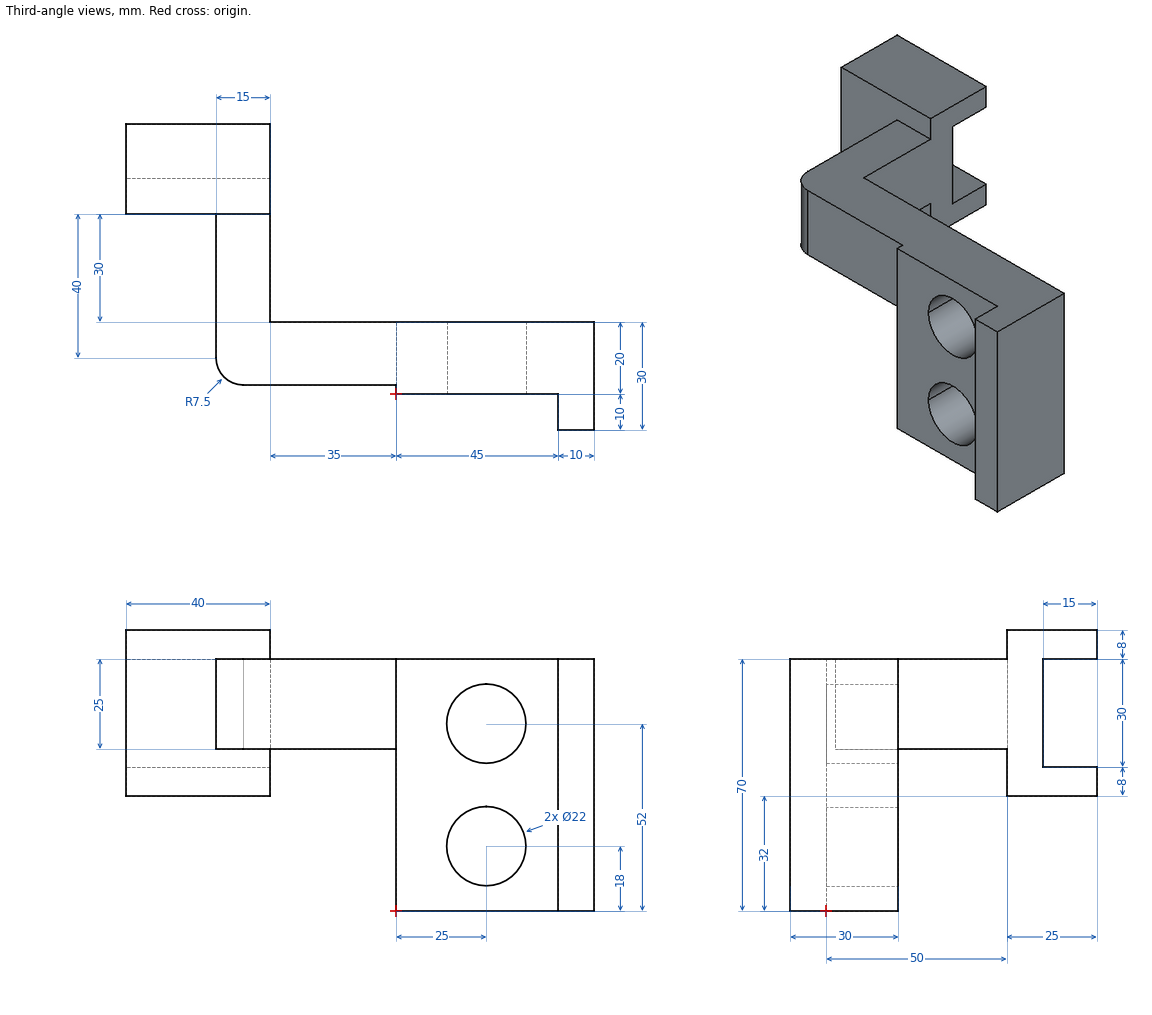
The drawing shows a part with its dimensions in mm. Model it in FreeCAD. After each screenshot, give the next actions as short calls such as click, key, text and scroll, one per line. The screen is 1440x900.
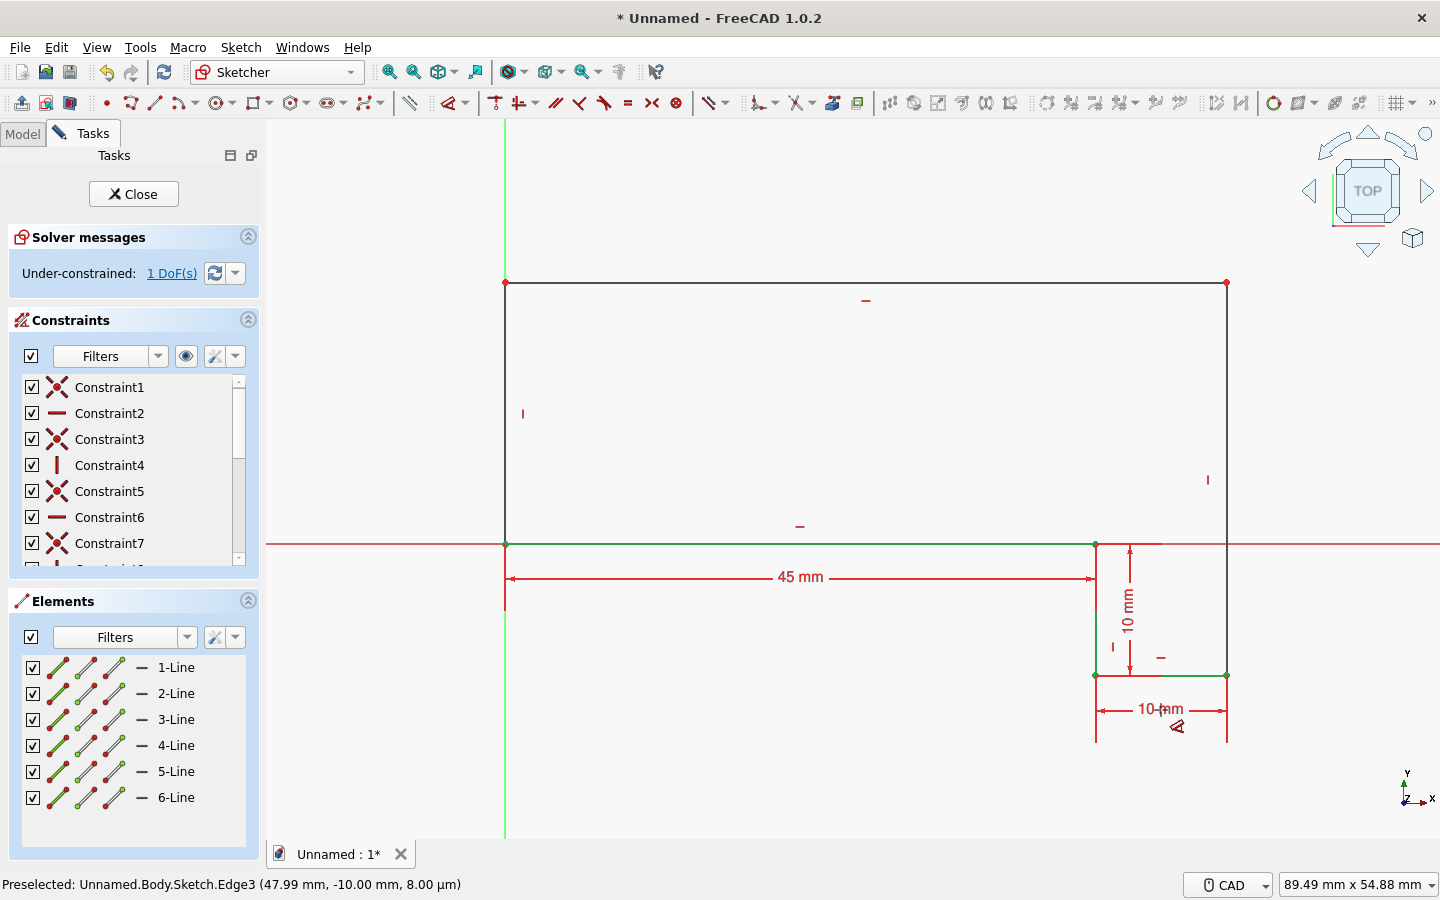
click(1227, 558)
click(1261, 479)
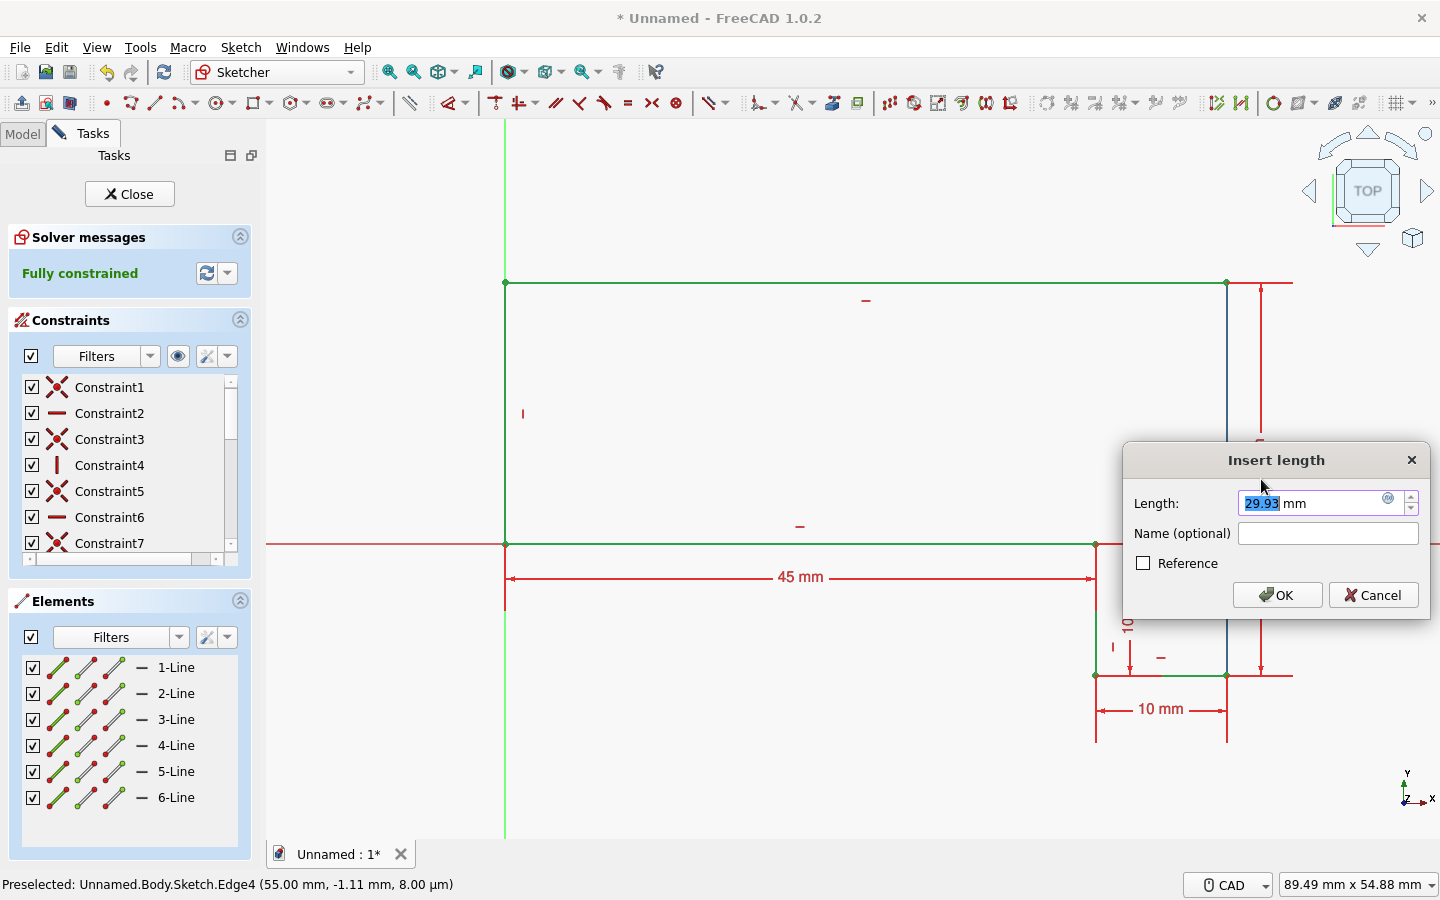
text(30)
key(Return)
key(Escape)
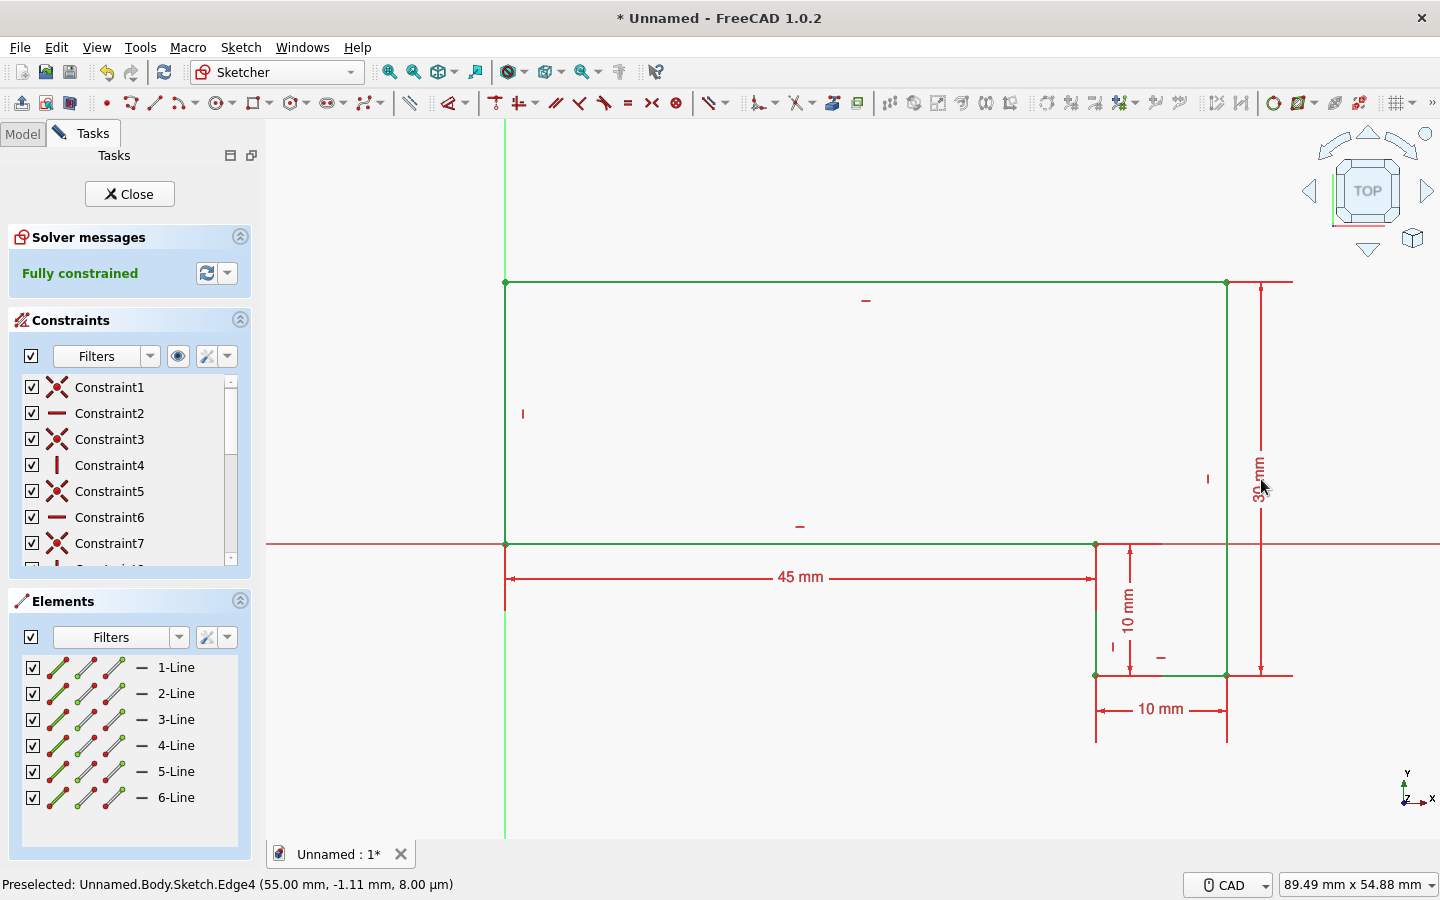
click(130, 194)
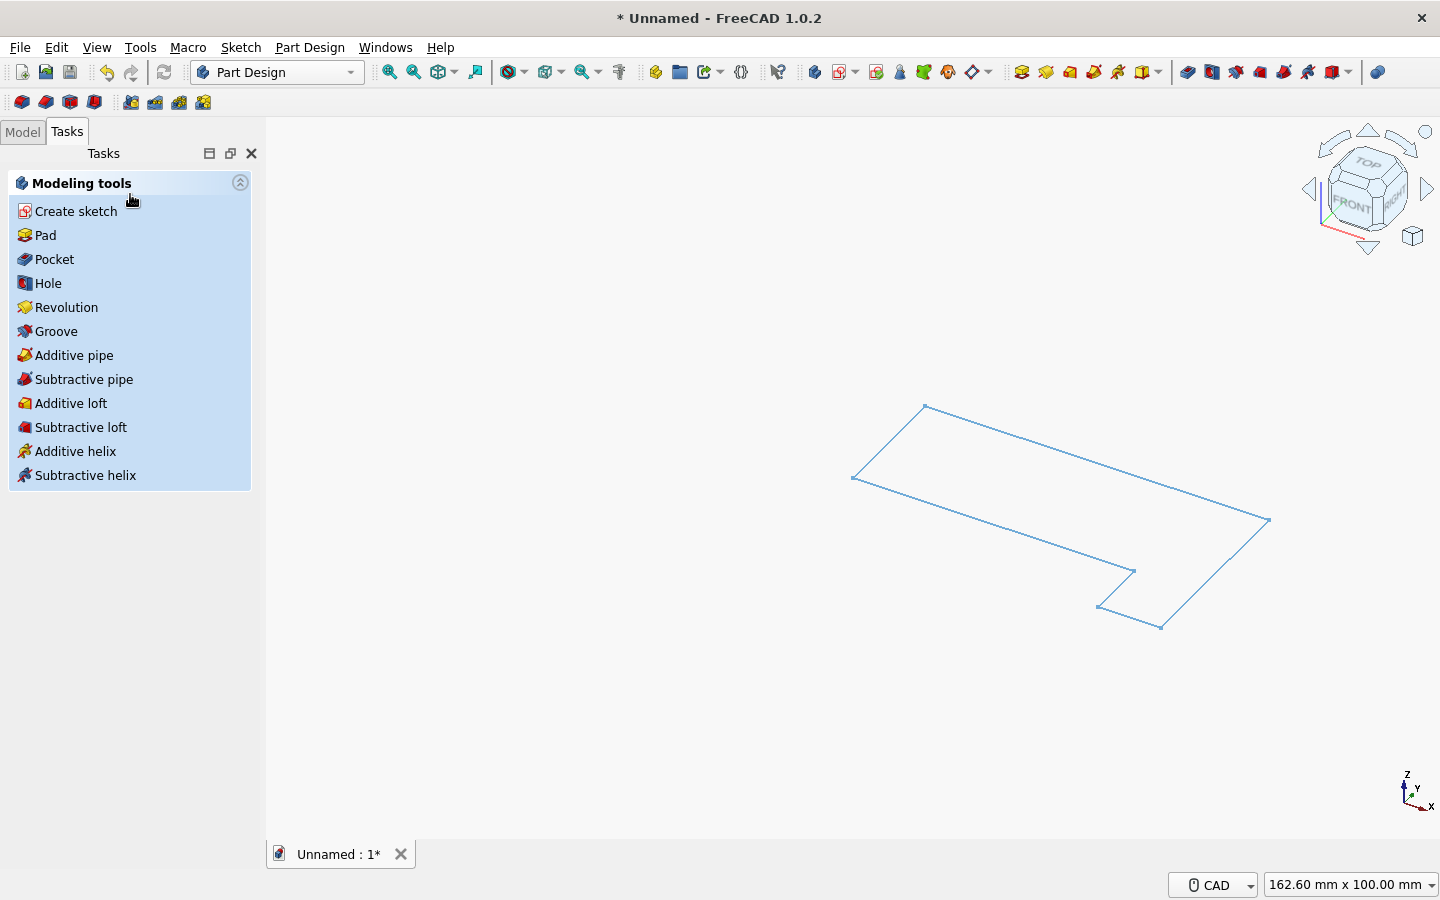
click(1022, 72)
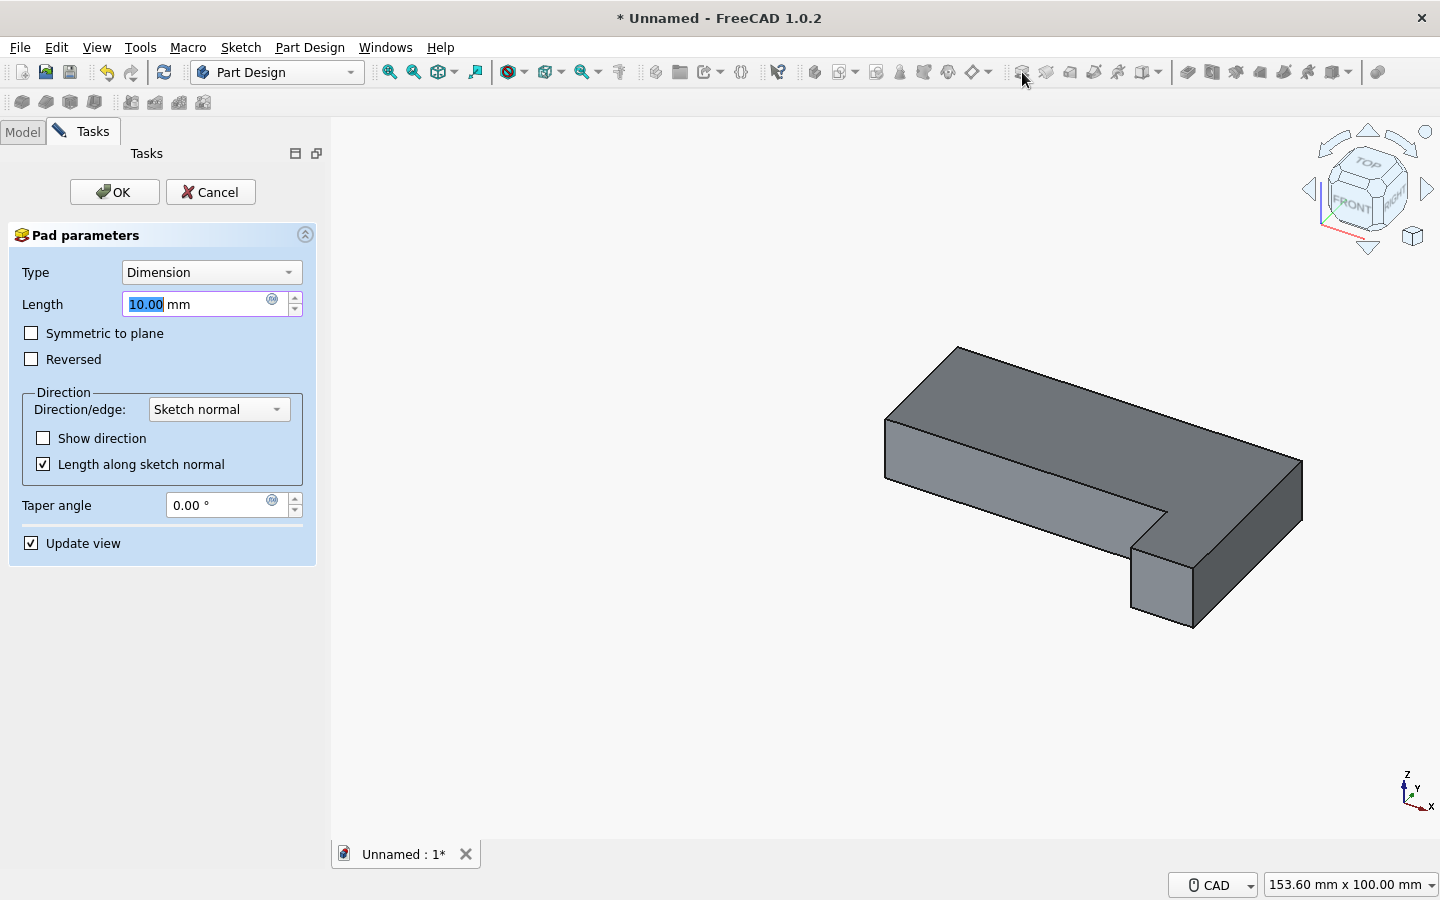
text(70)
key(Tab)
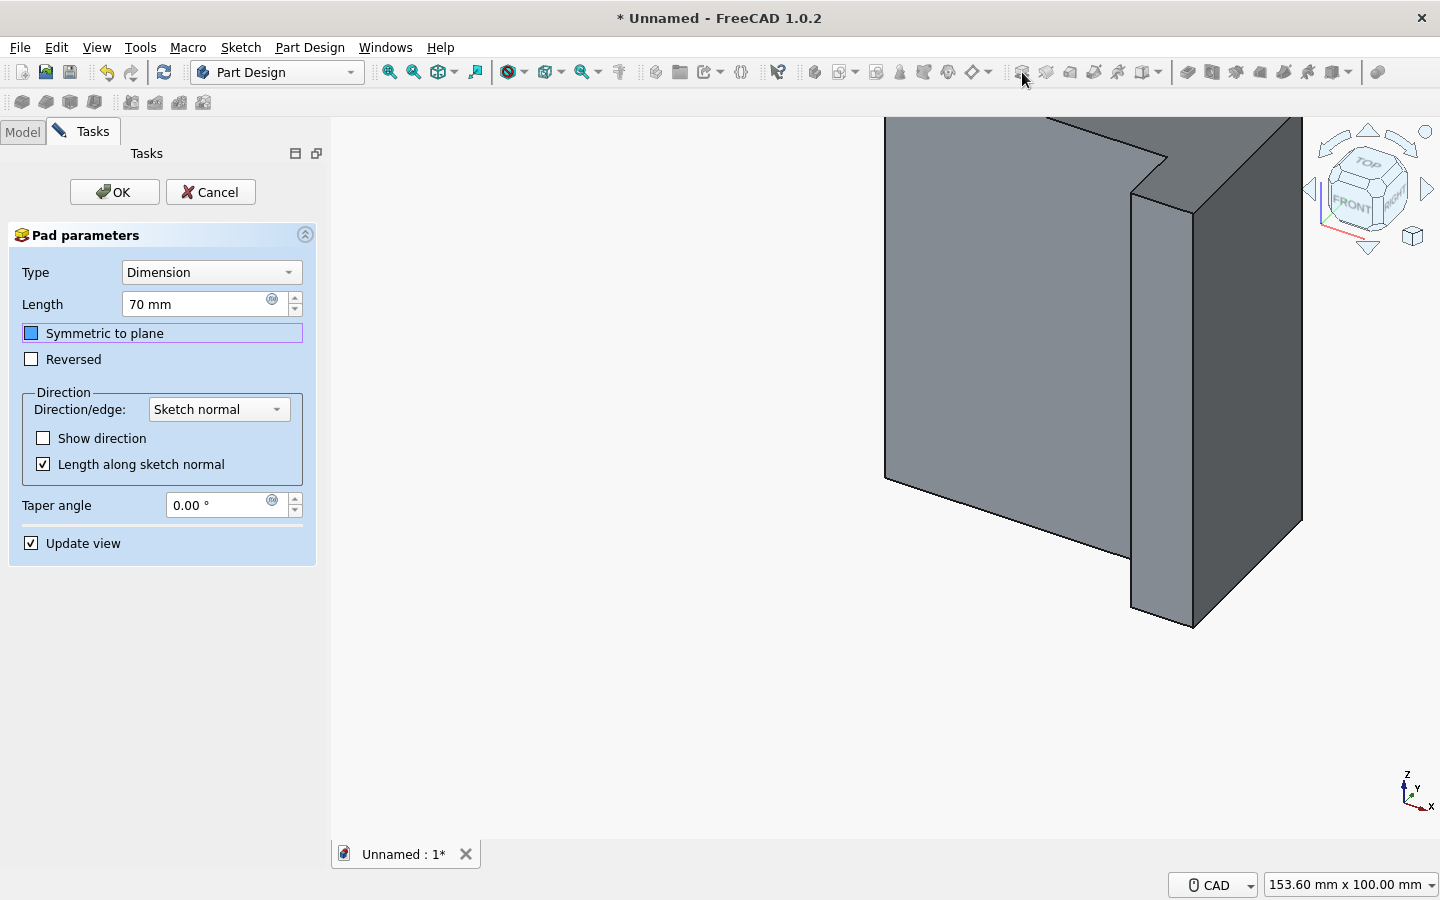
click(115, 192)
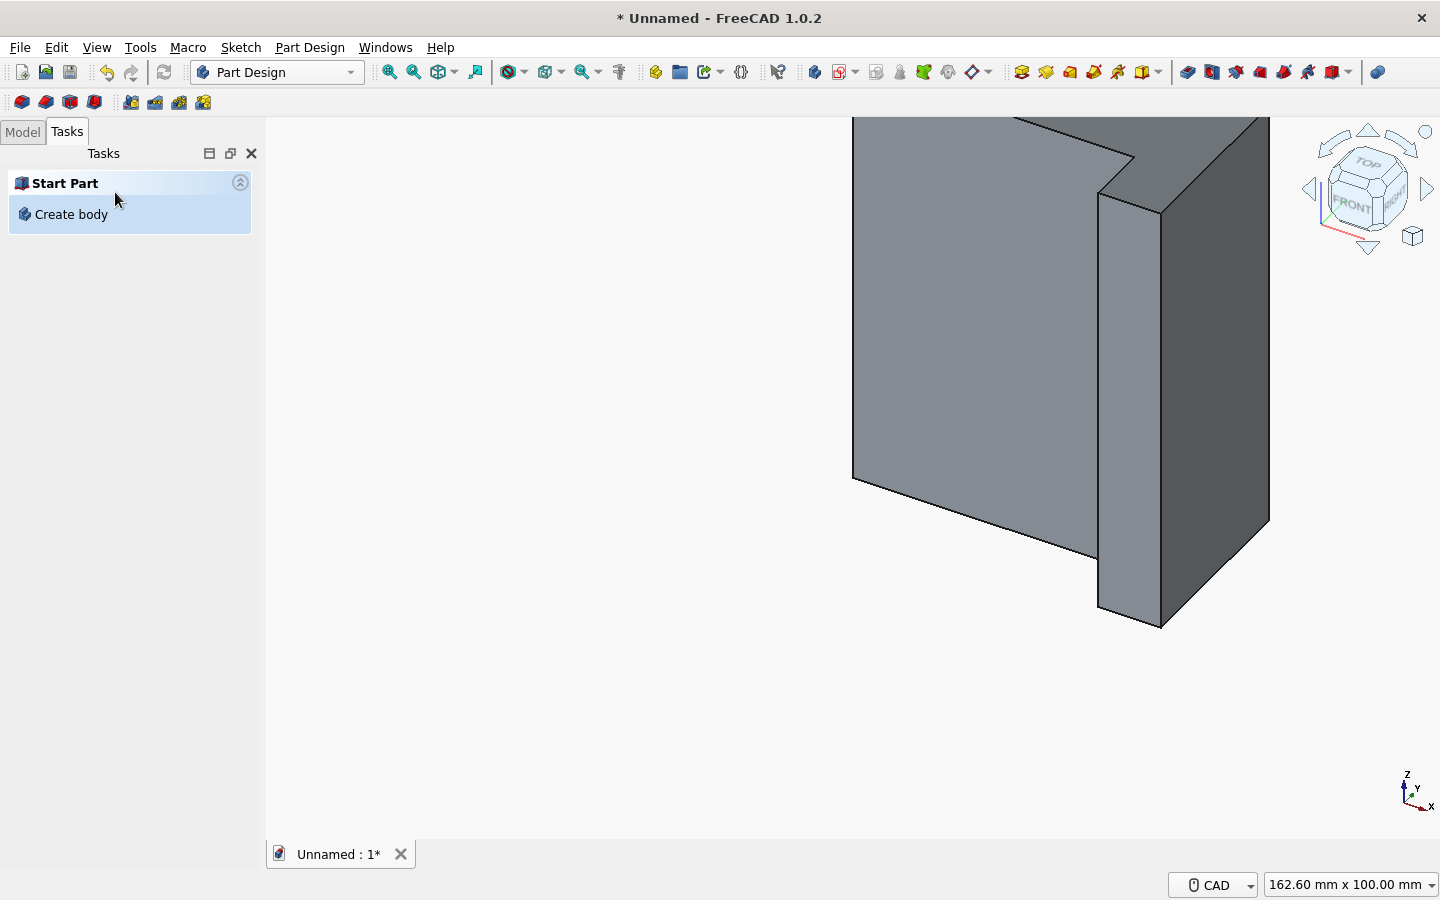
key(v)
key(f)